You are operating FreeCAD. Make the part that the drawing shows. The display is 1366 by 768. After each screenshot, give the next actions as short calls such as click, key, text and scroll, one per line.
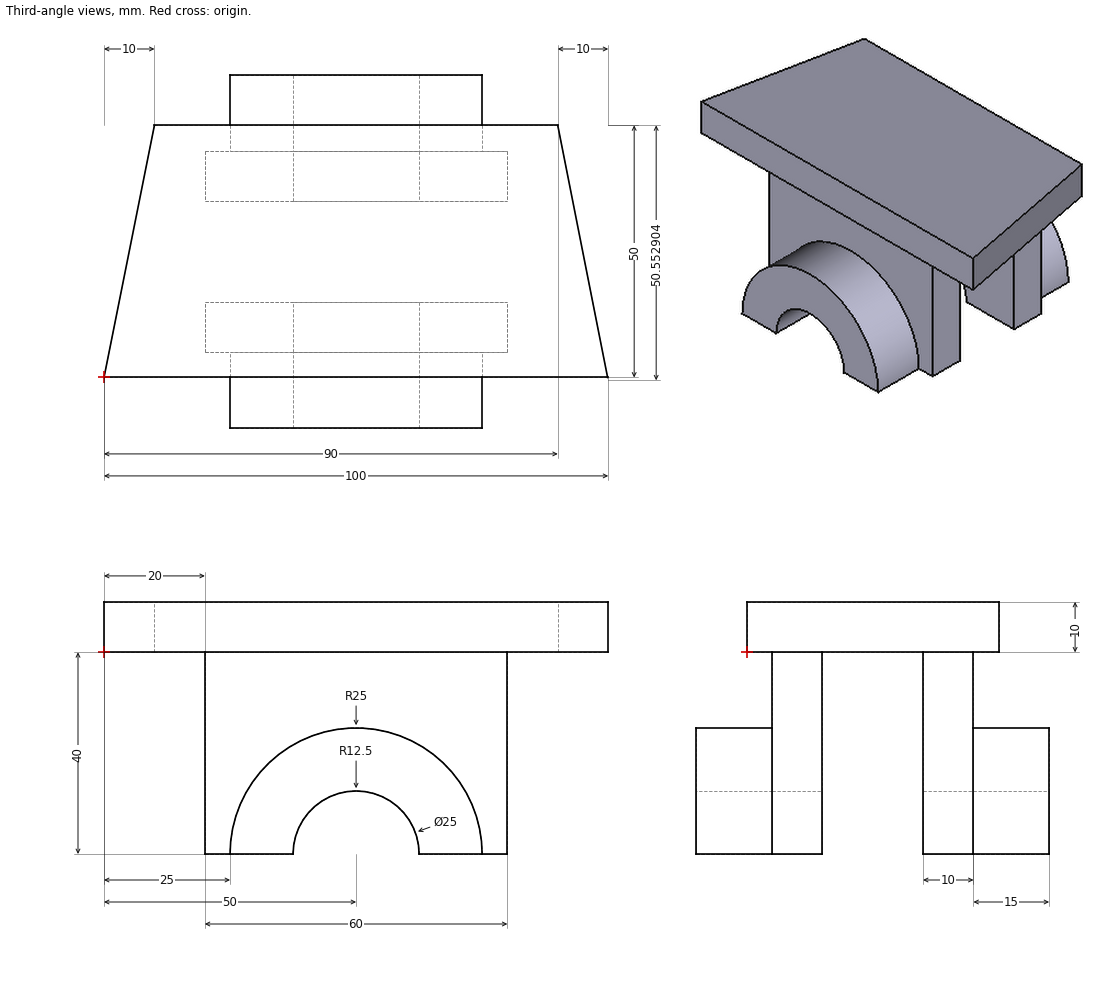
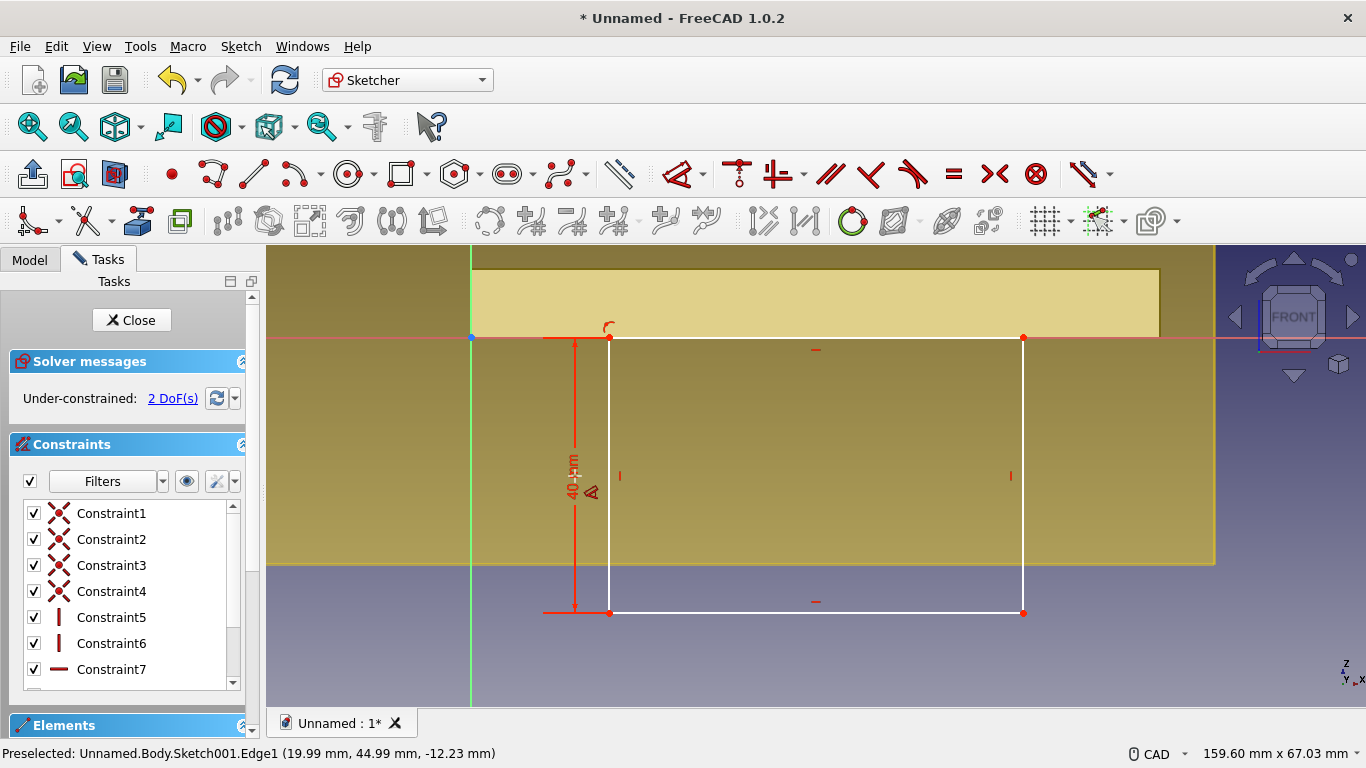
click(733, 613)
click(816, 647)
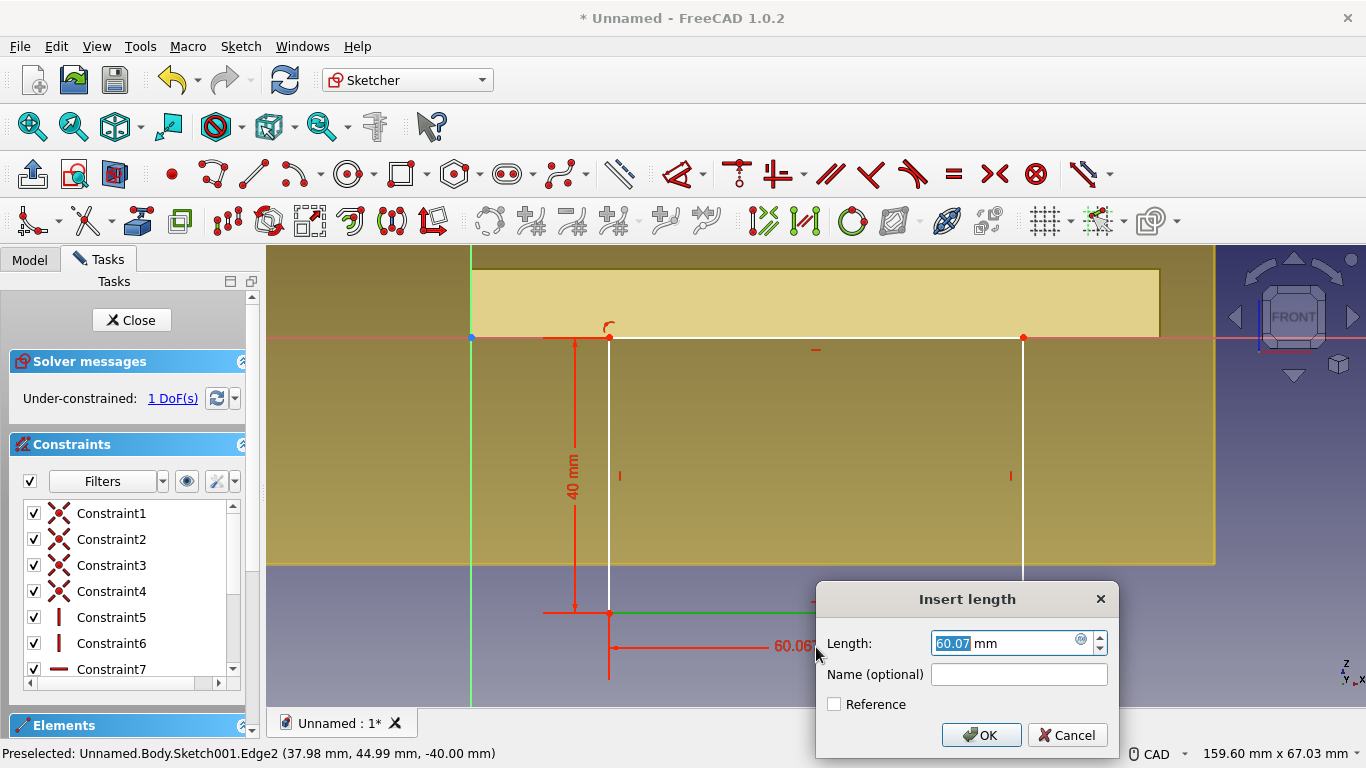
text(60)
key(Return)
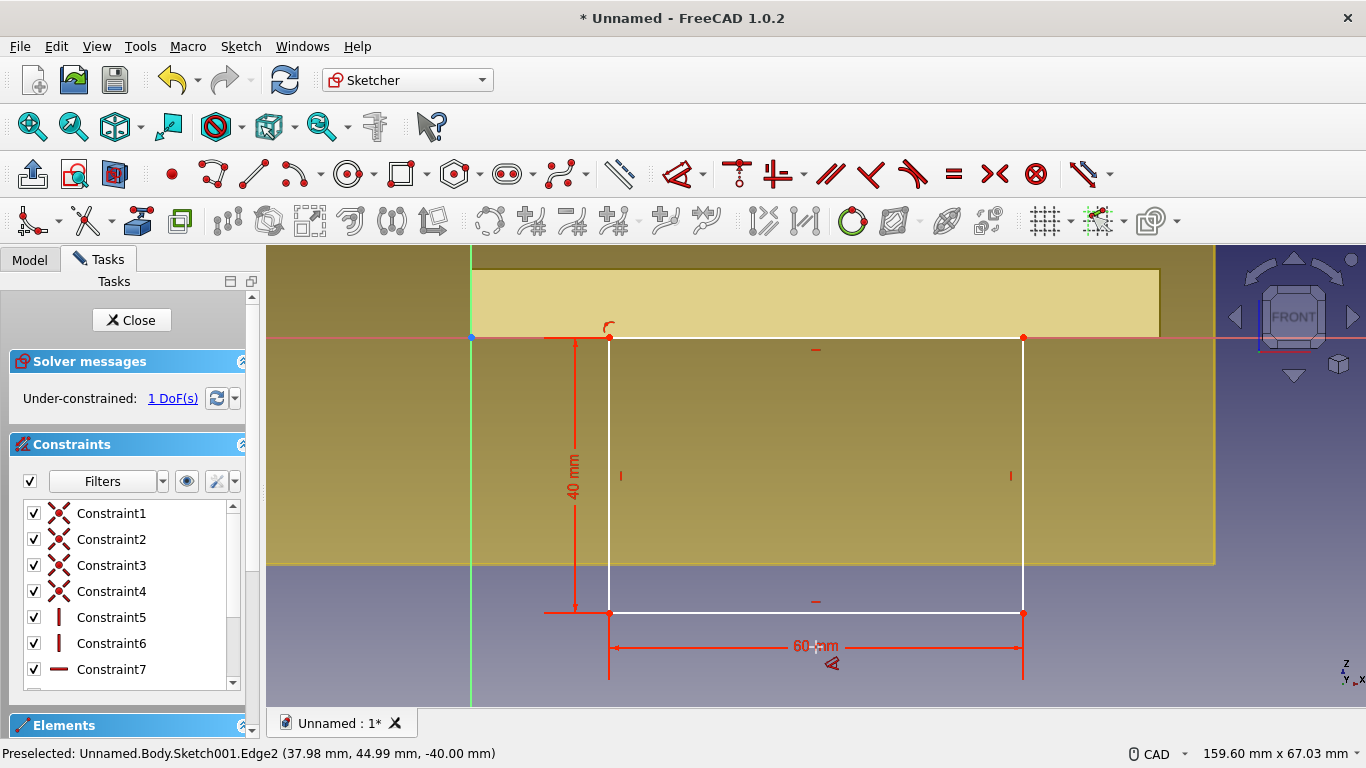
click(609, 338)
click(540, 304)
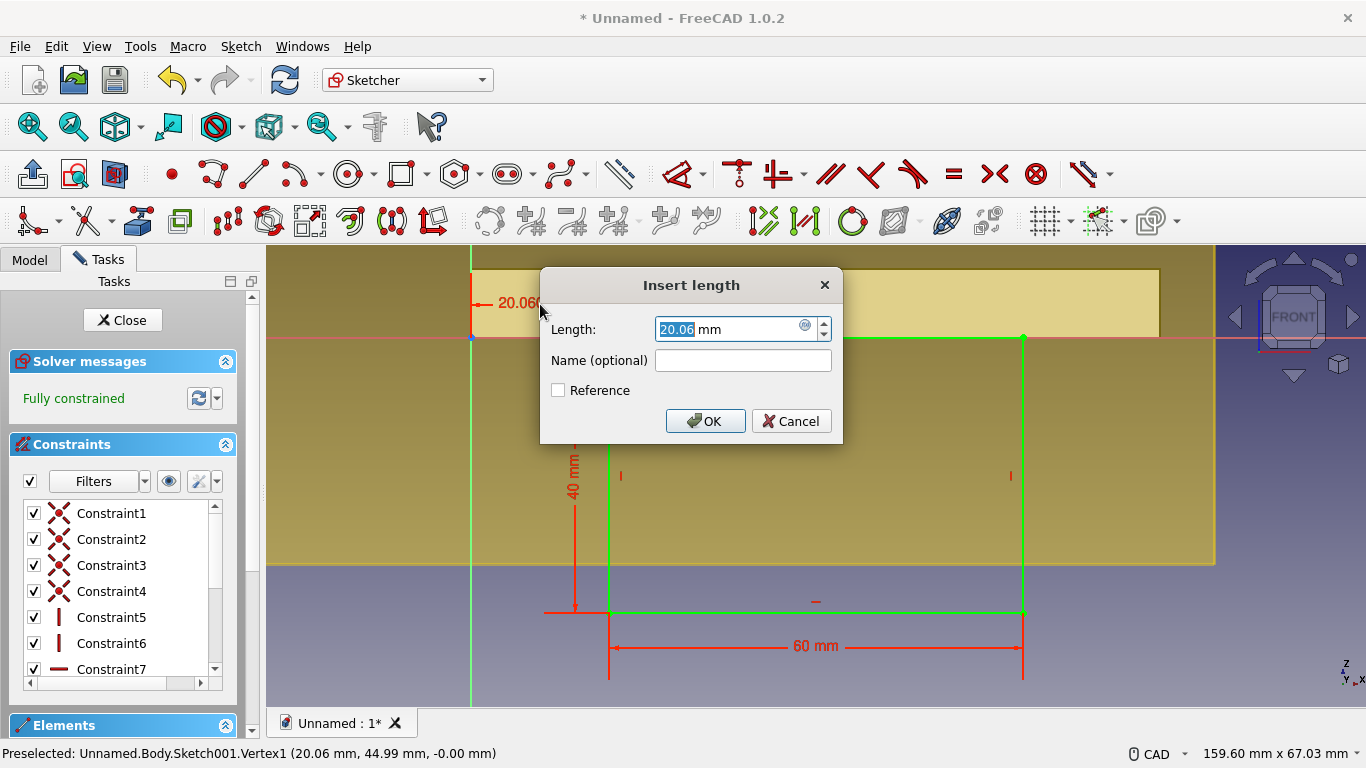
text(20)
key(Return)
key(Escape)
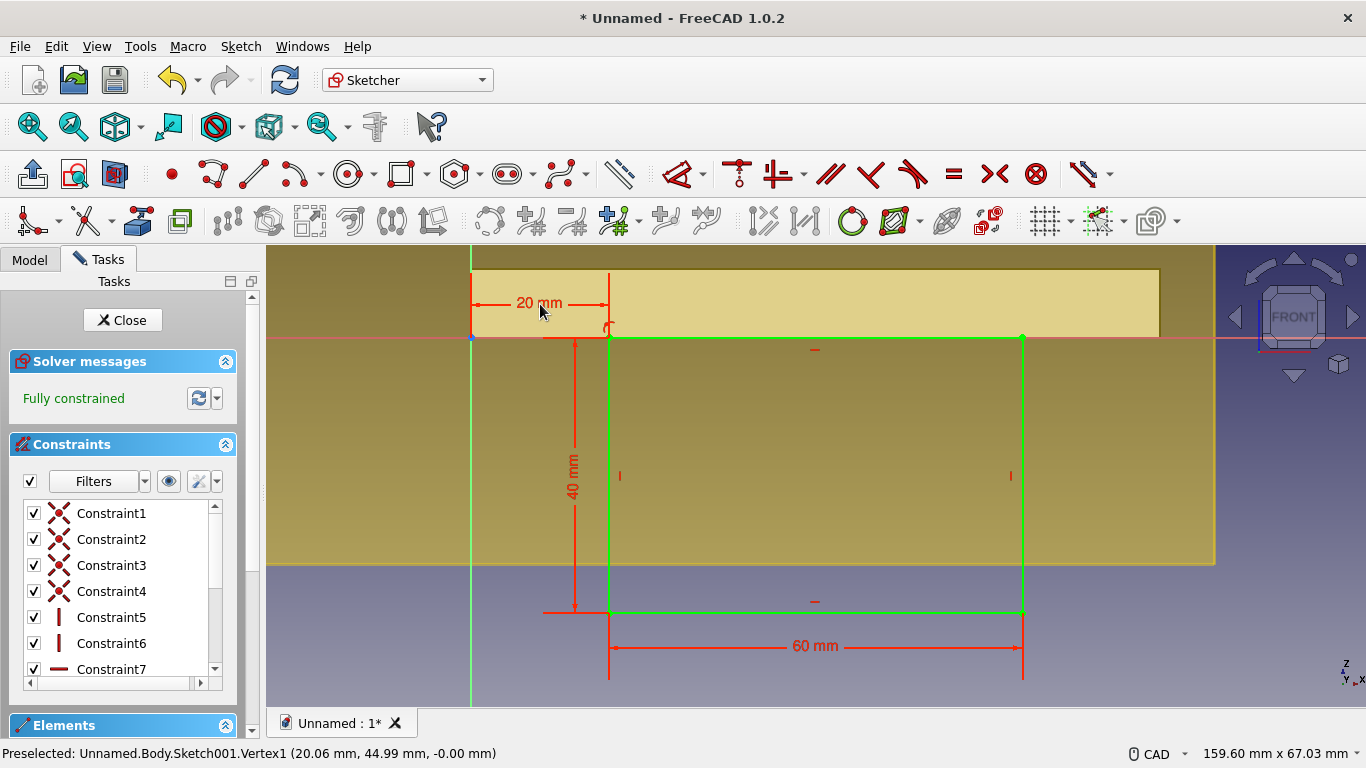
click(123, 320)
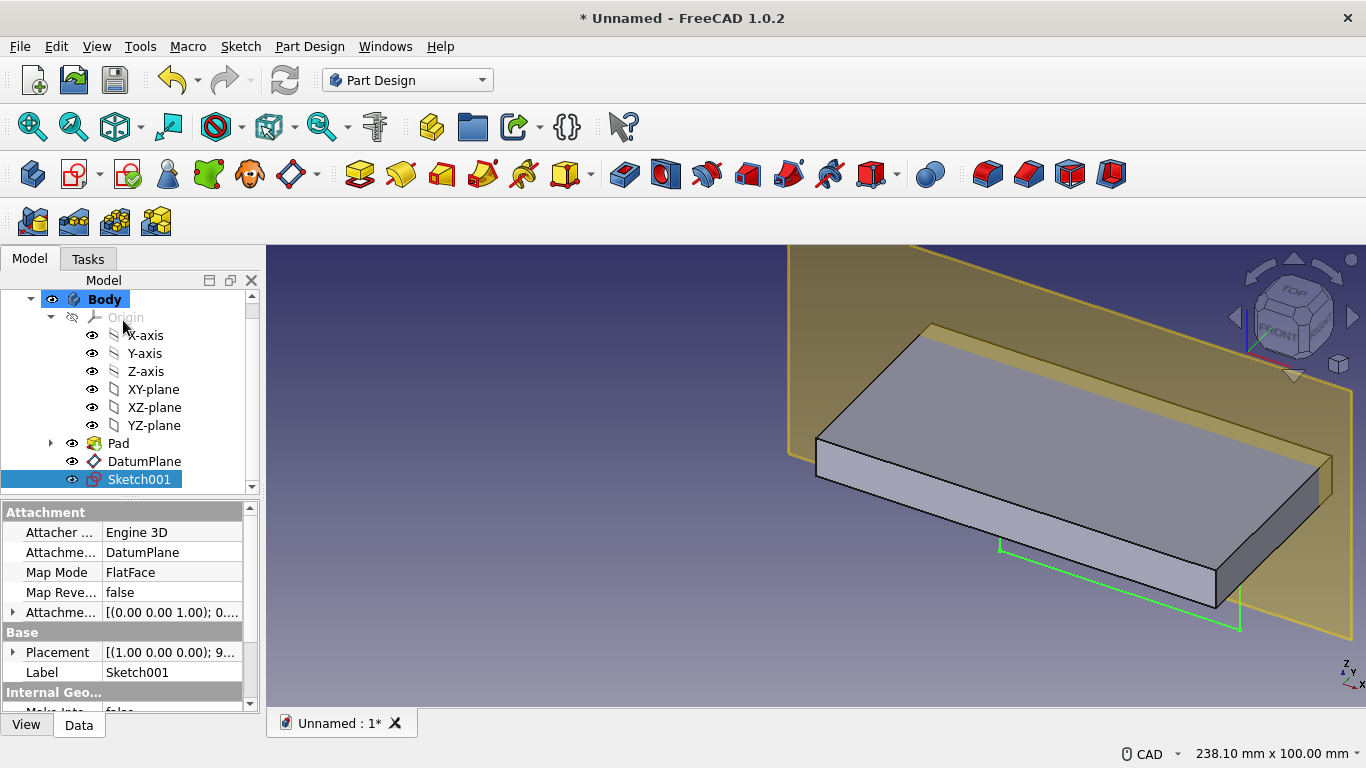
click(360, 174)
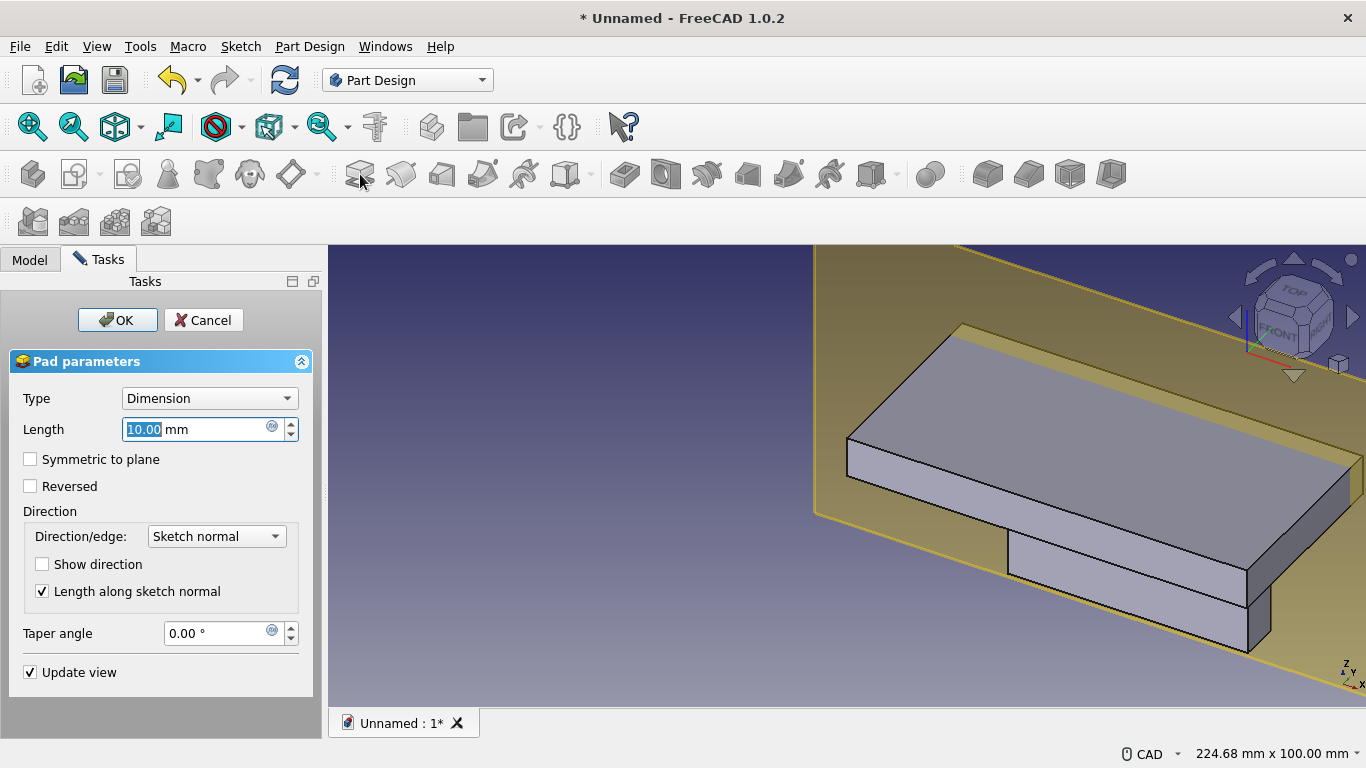
text(10)
key(Tab)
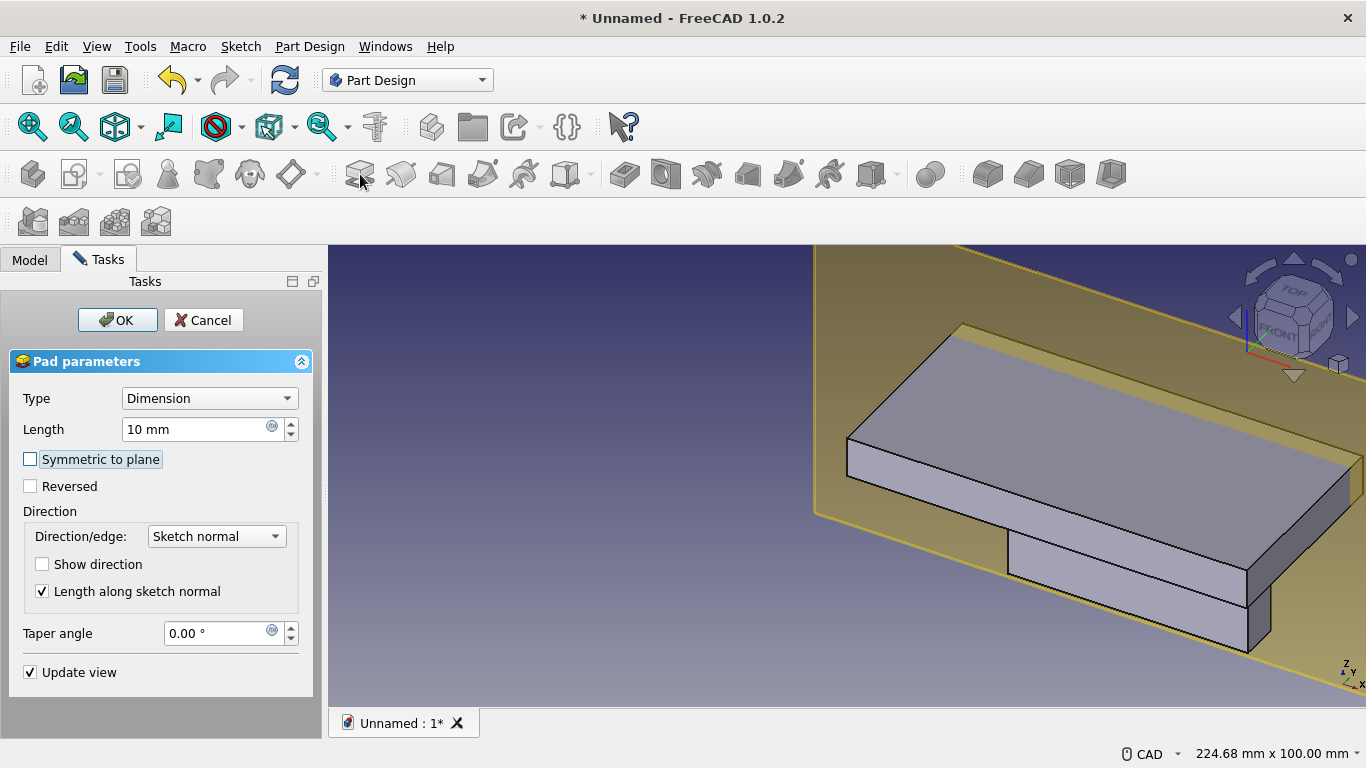
click(118, 320)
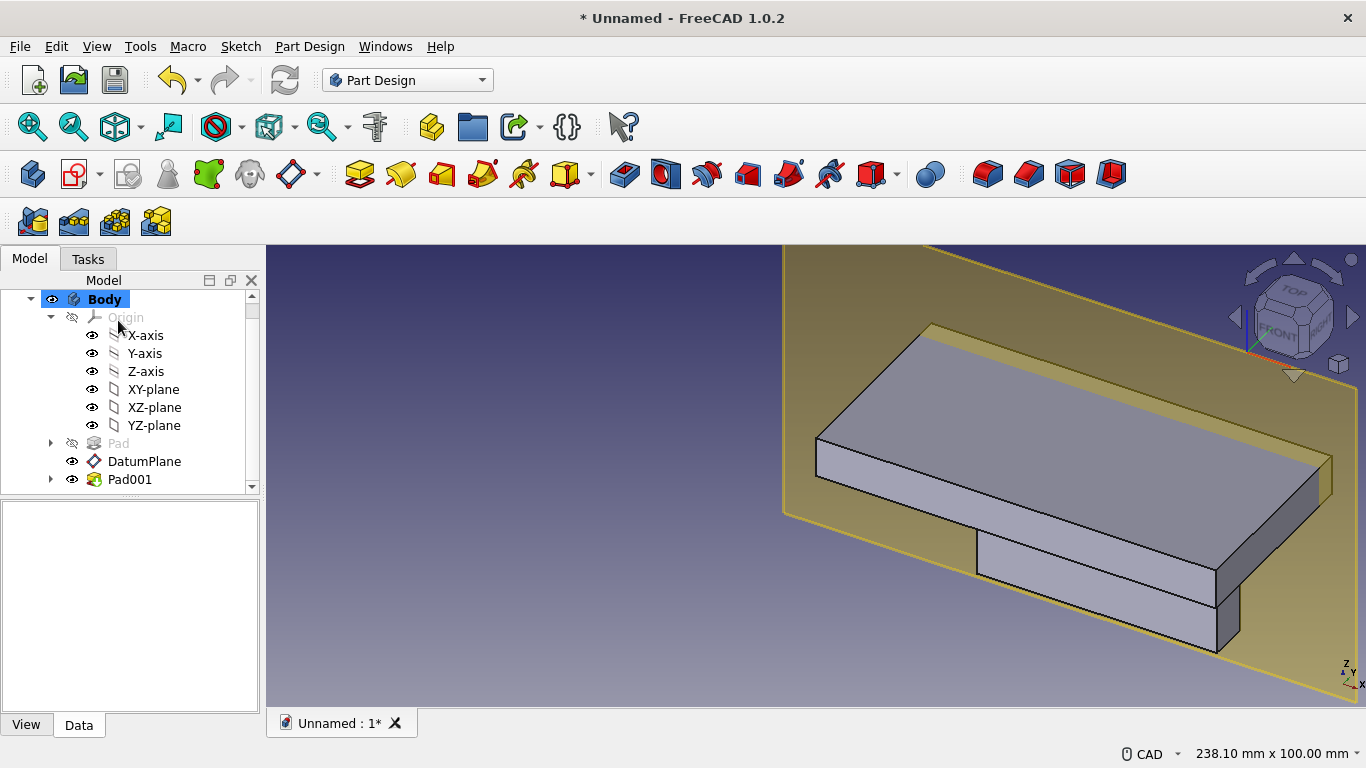
click(117, 461)
key(space)